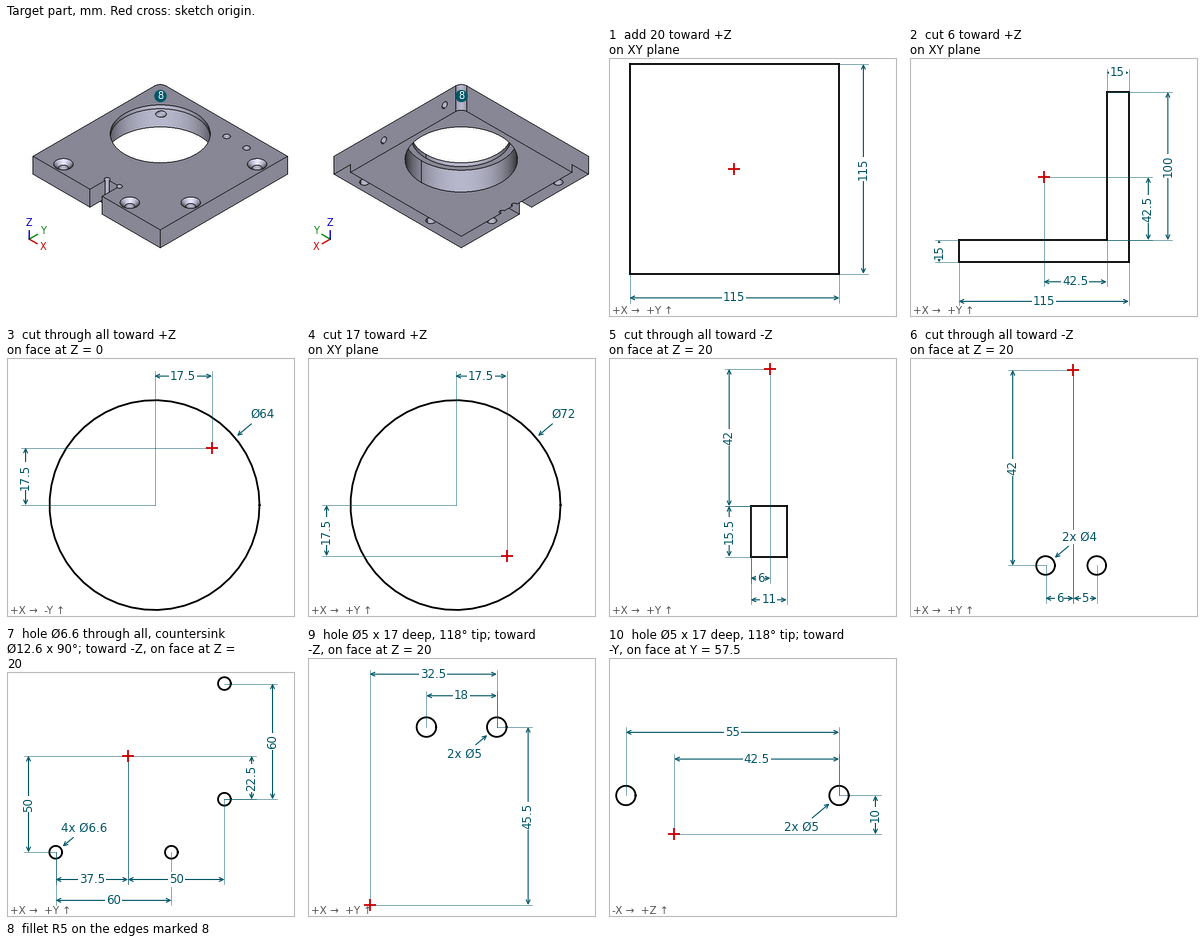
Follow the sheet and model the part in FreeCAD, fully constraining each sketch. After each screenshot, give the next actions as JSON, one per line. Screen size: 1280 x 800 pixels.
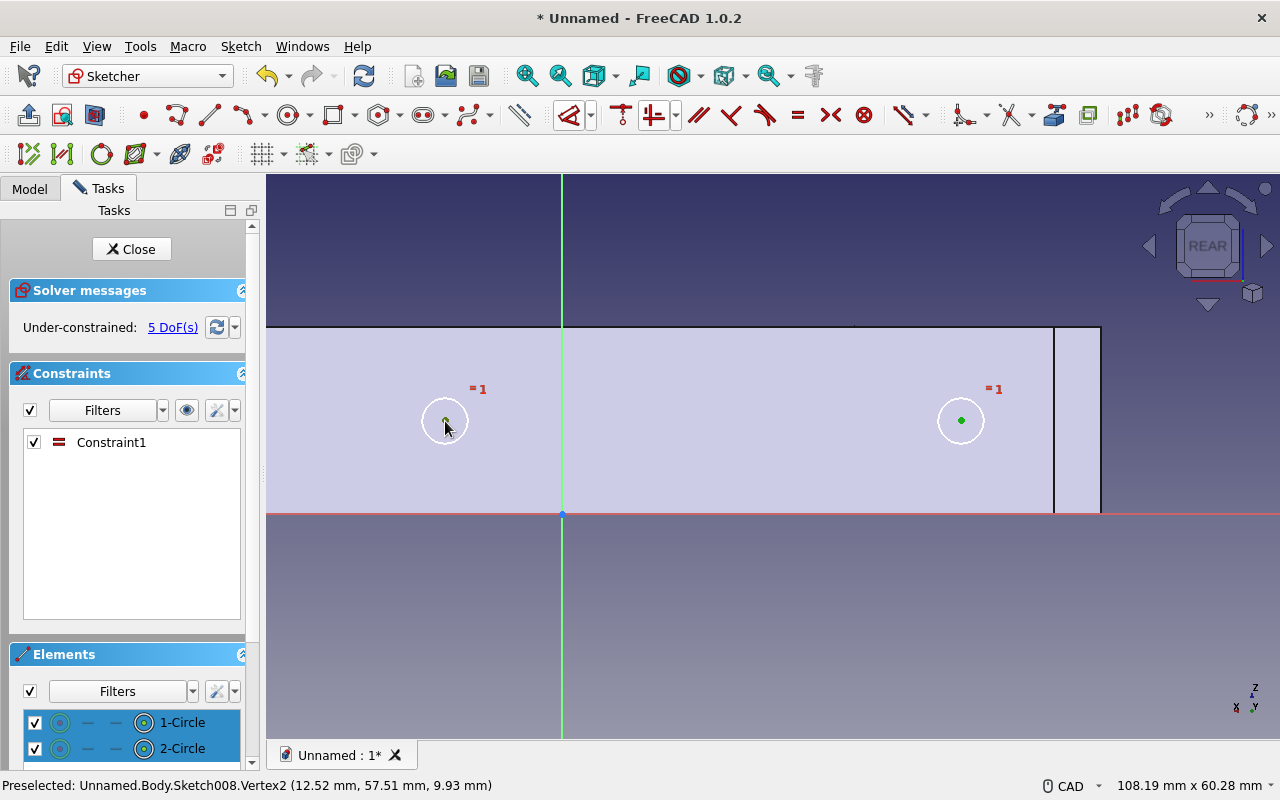
{"action": "key", "text": "h"}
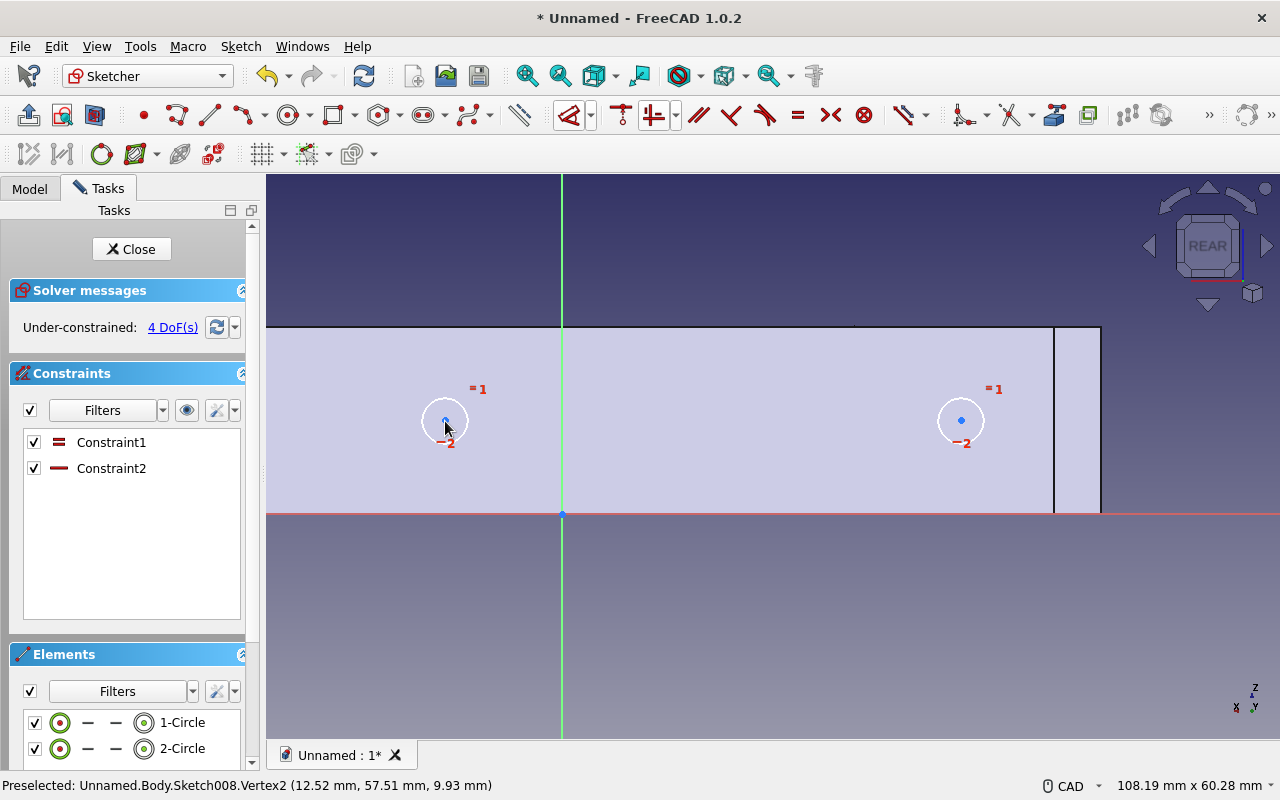
{"action": "left_click", "coordinate": [977, 405]}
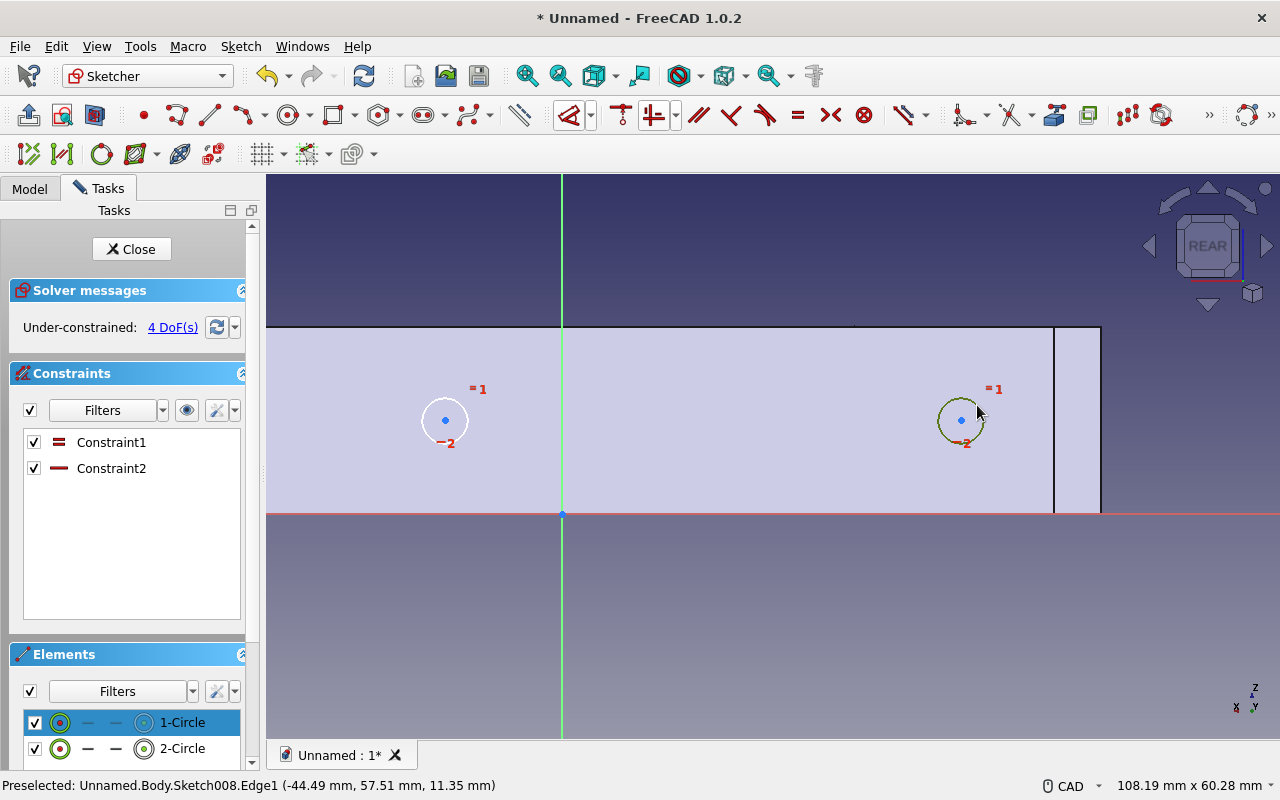
{"action": "key", "text": "k o"}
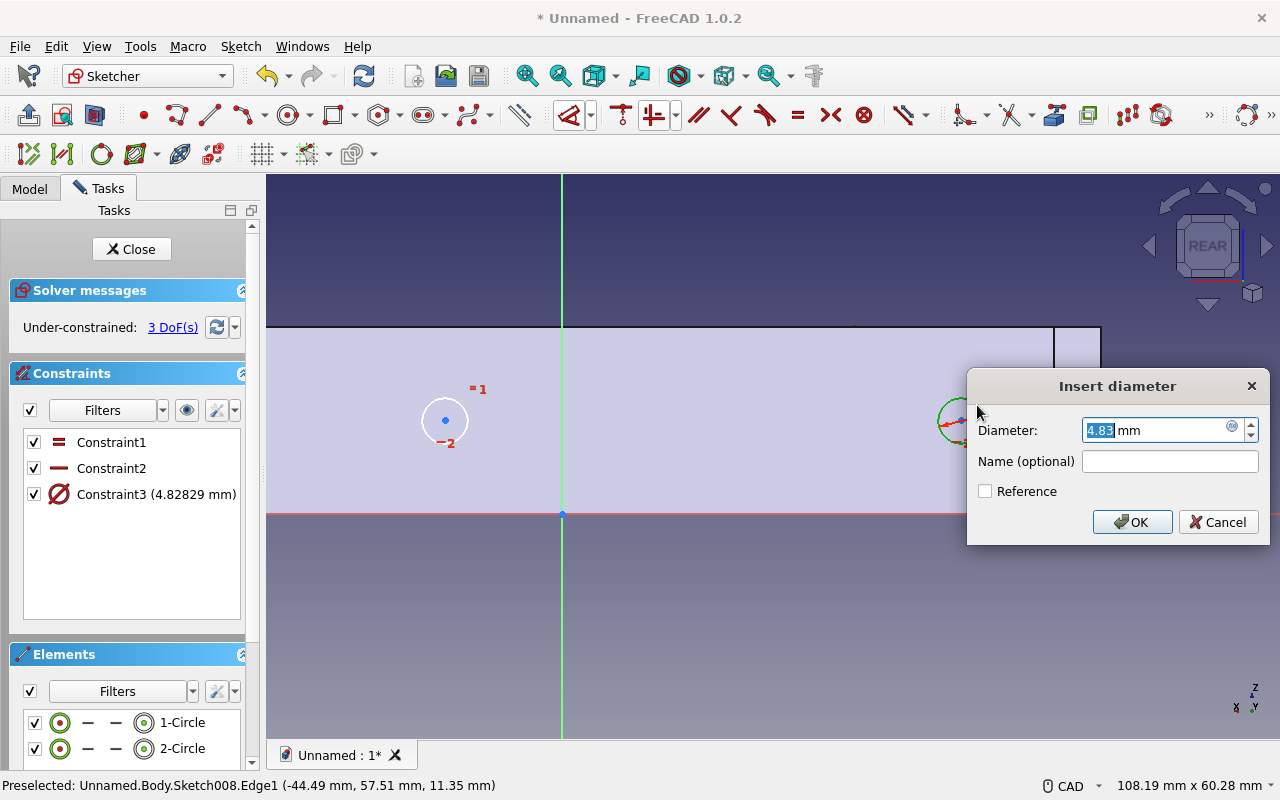
{"action": "type", "text": "5"}
{"action": "key", "text": "Return"}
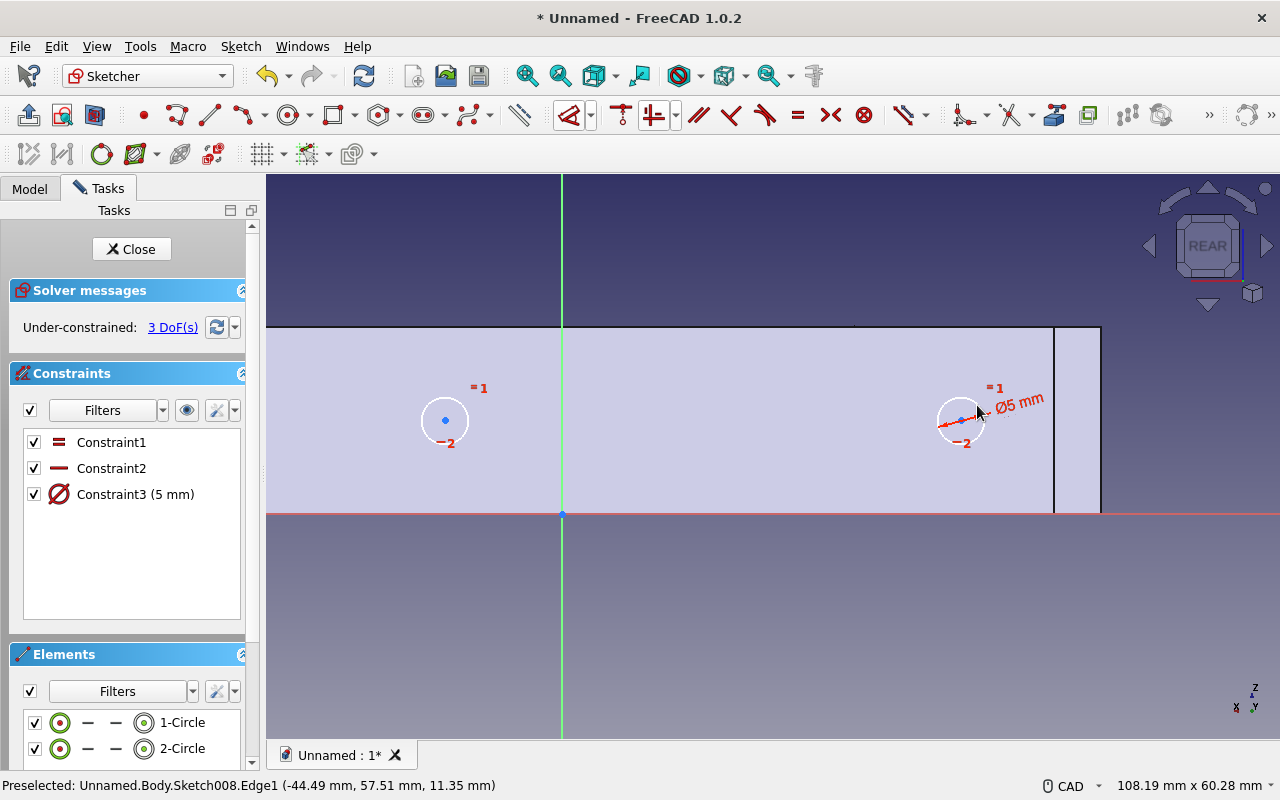
{"action": "left_click", "coordinate": [961, 421]}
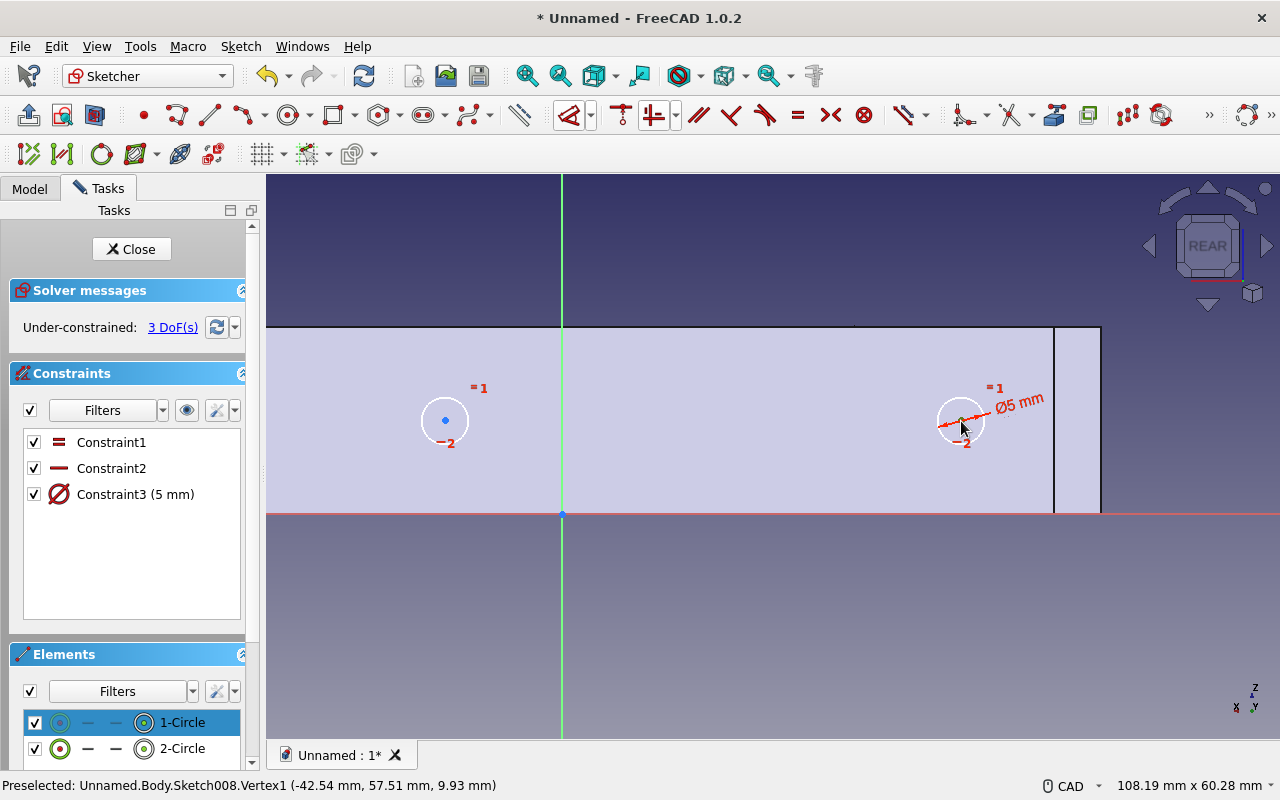
{"action": "key", "text": "i"}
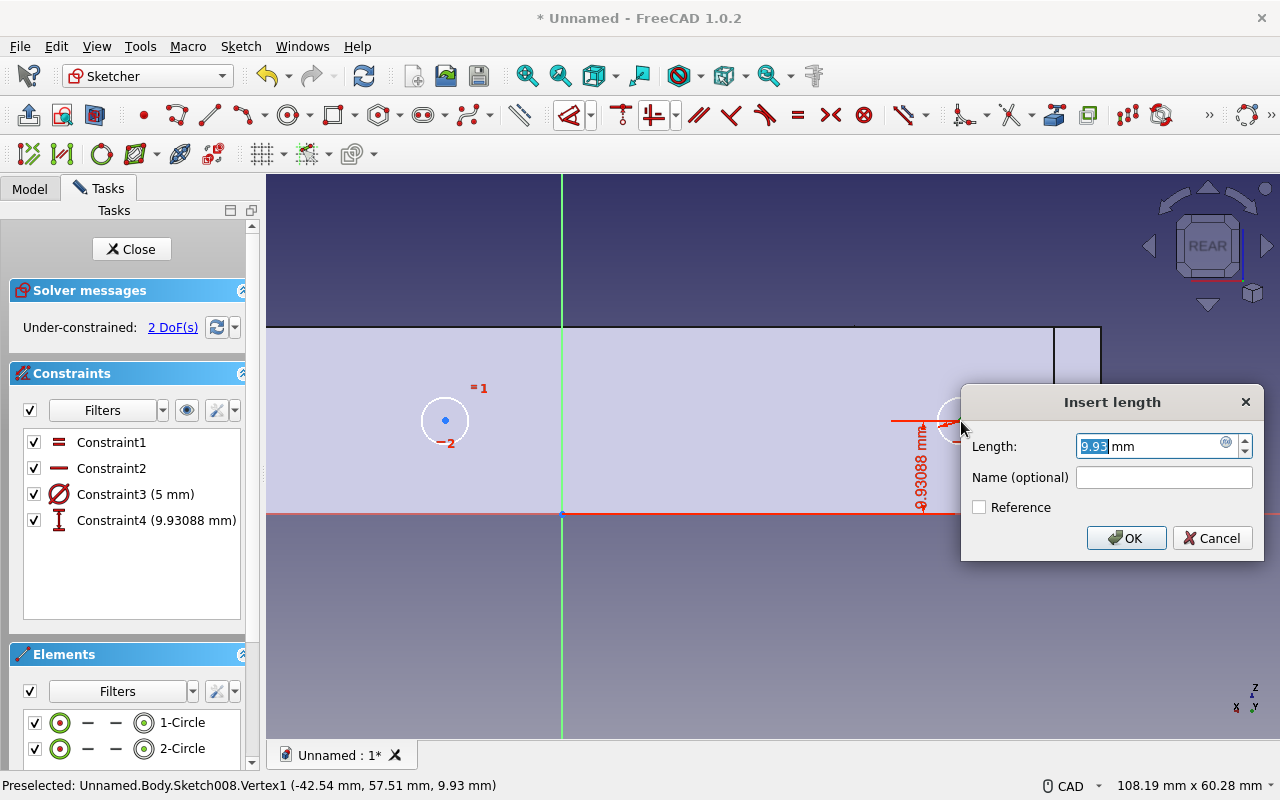
{"action": "type", "text": "10"}
{"action": "key", "text": "Return"}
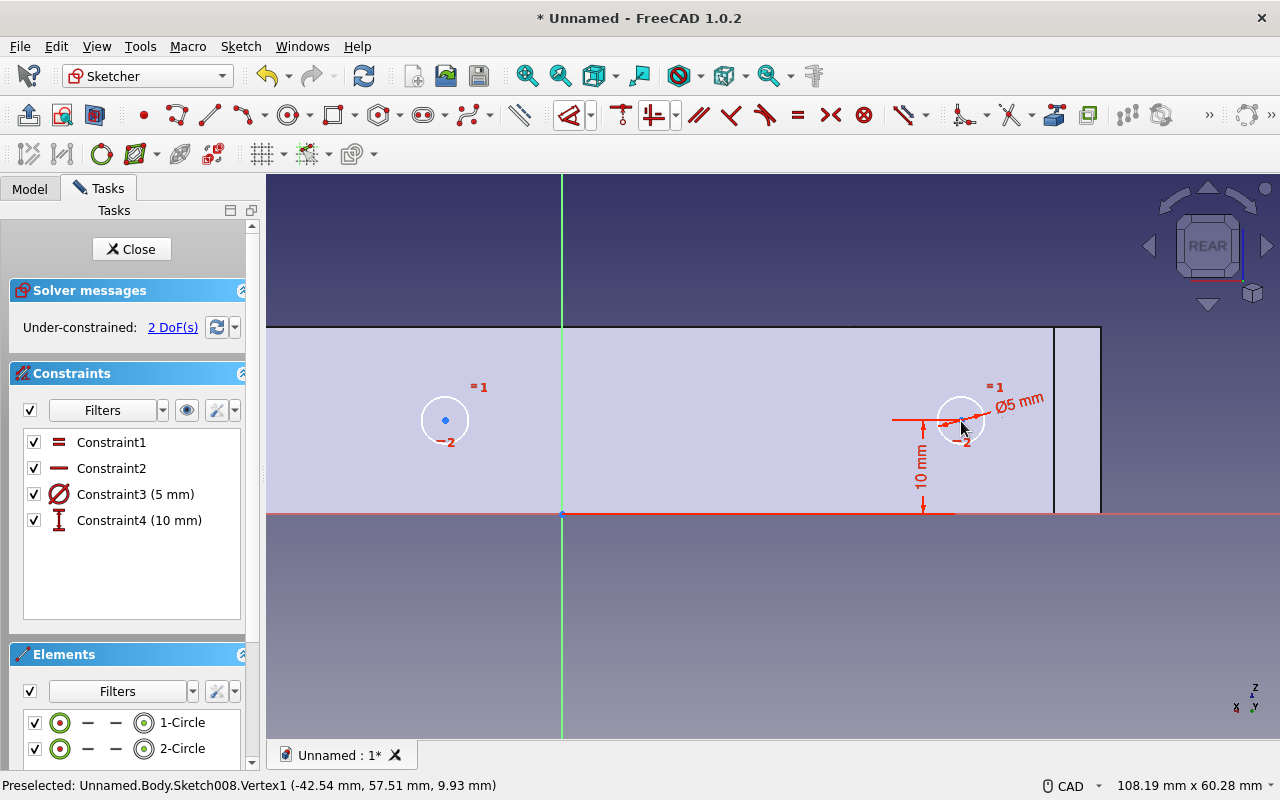
{"action": "left_click", "coordinate": [961, 420]}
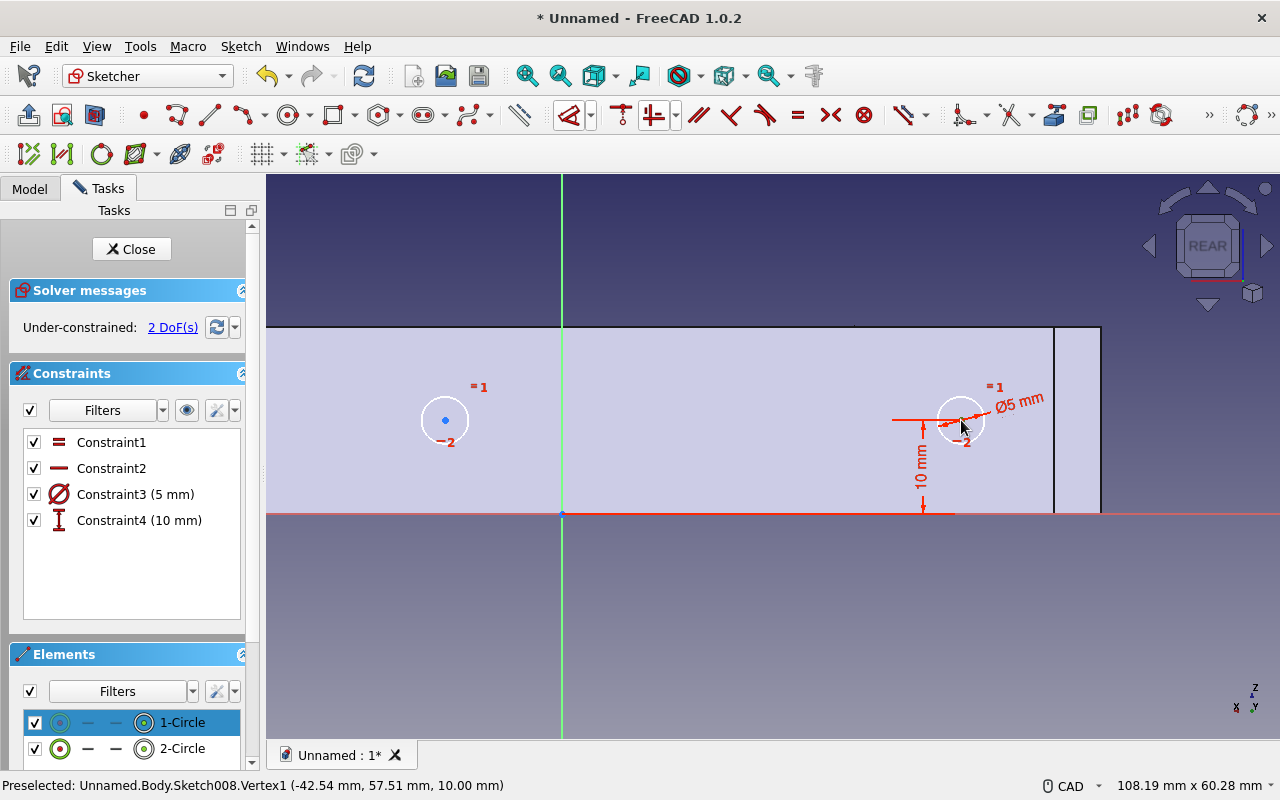
{"action": "left_click", "coordinate": [445, 420]}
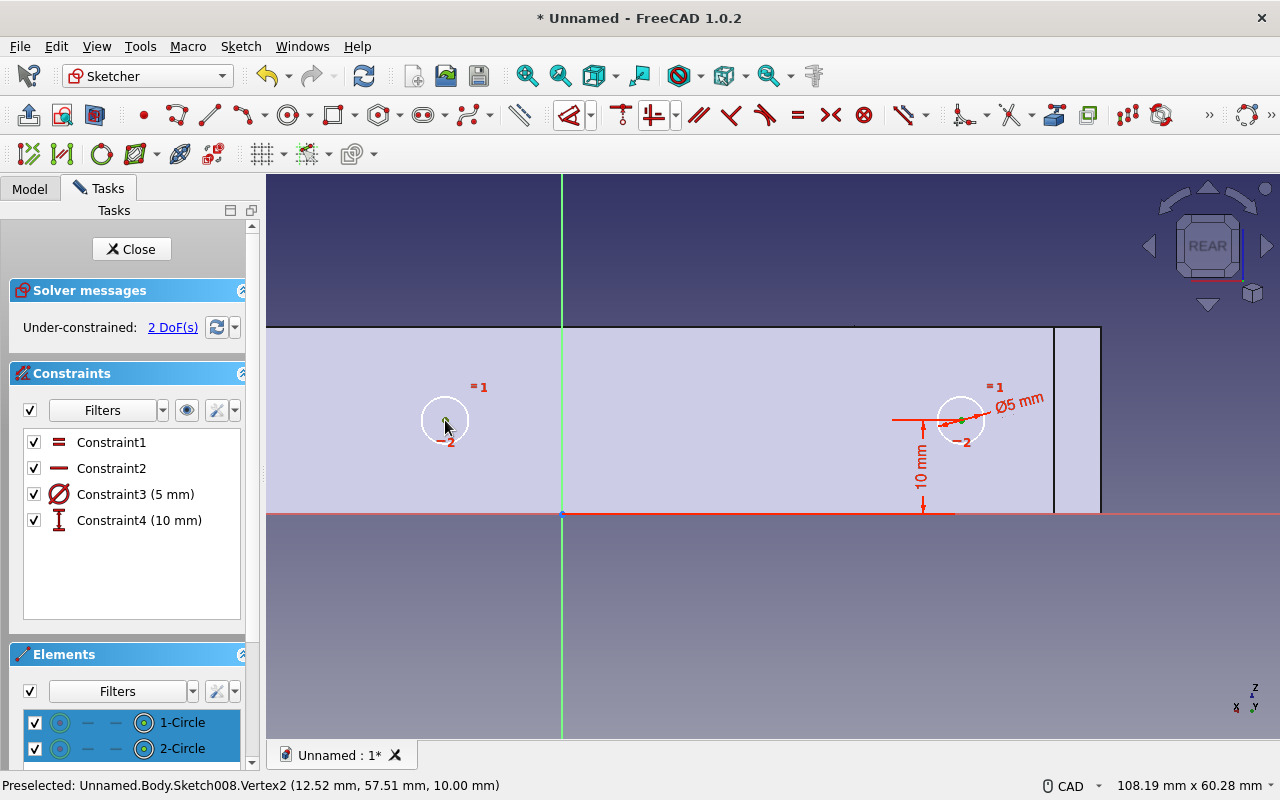
{"action": "left_click", "coordinate": [590, 116]}